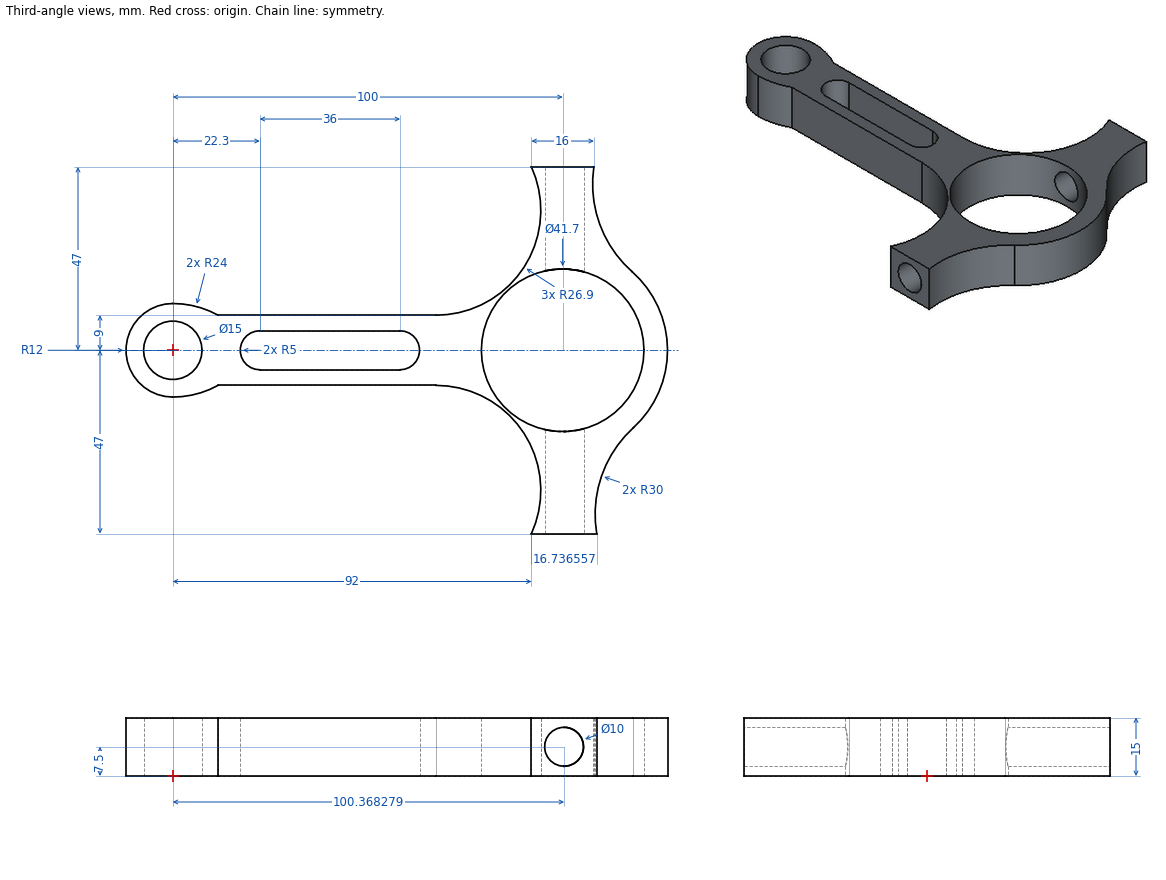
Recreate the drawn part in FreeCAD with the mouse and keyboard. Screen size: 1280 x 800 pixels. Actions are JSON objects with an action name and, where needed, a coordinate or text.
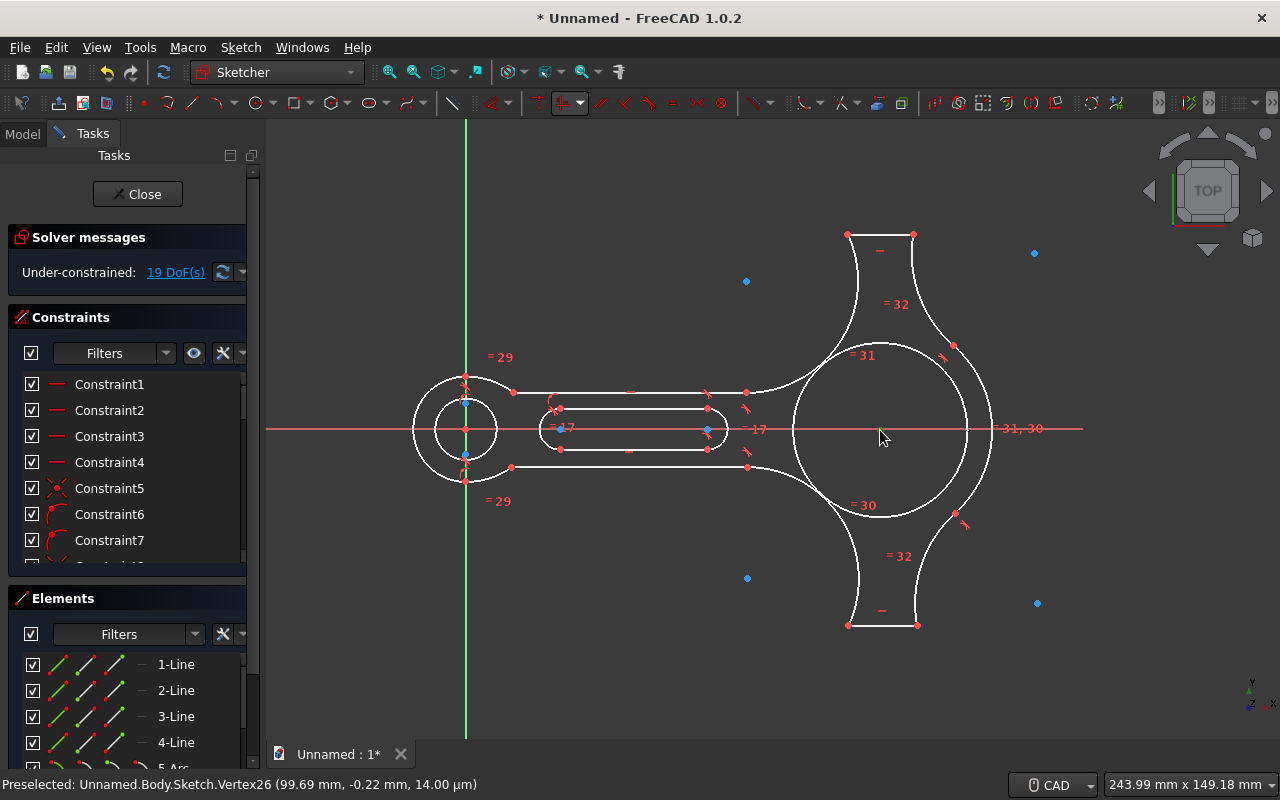
{"action": "left_click", "coordinate": [353, 429]}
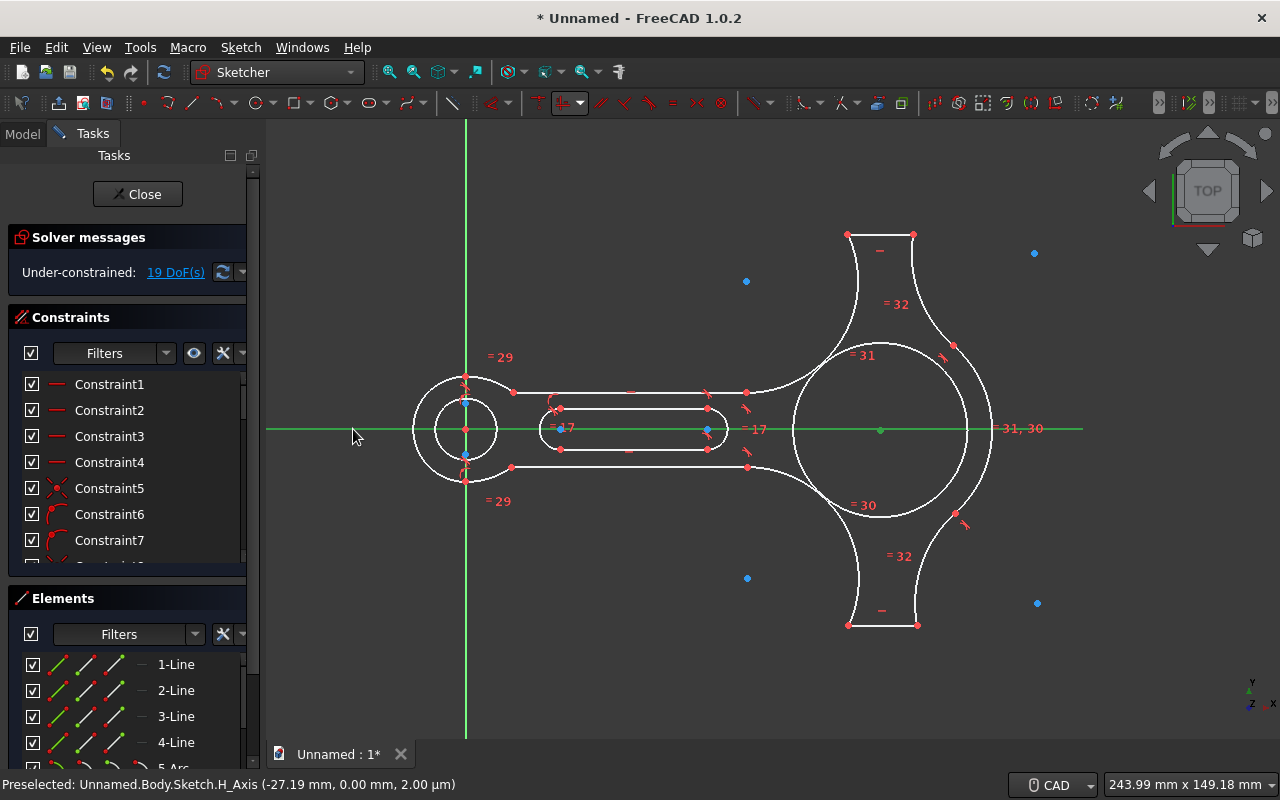
{"action": "left_click", "coordinate": [538, 104]}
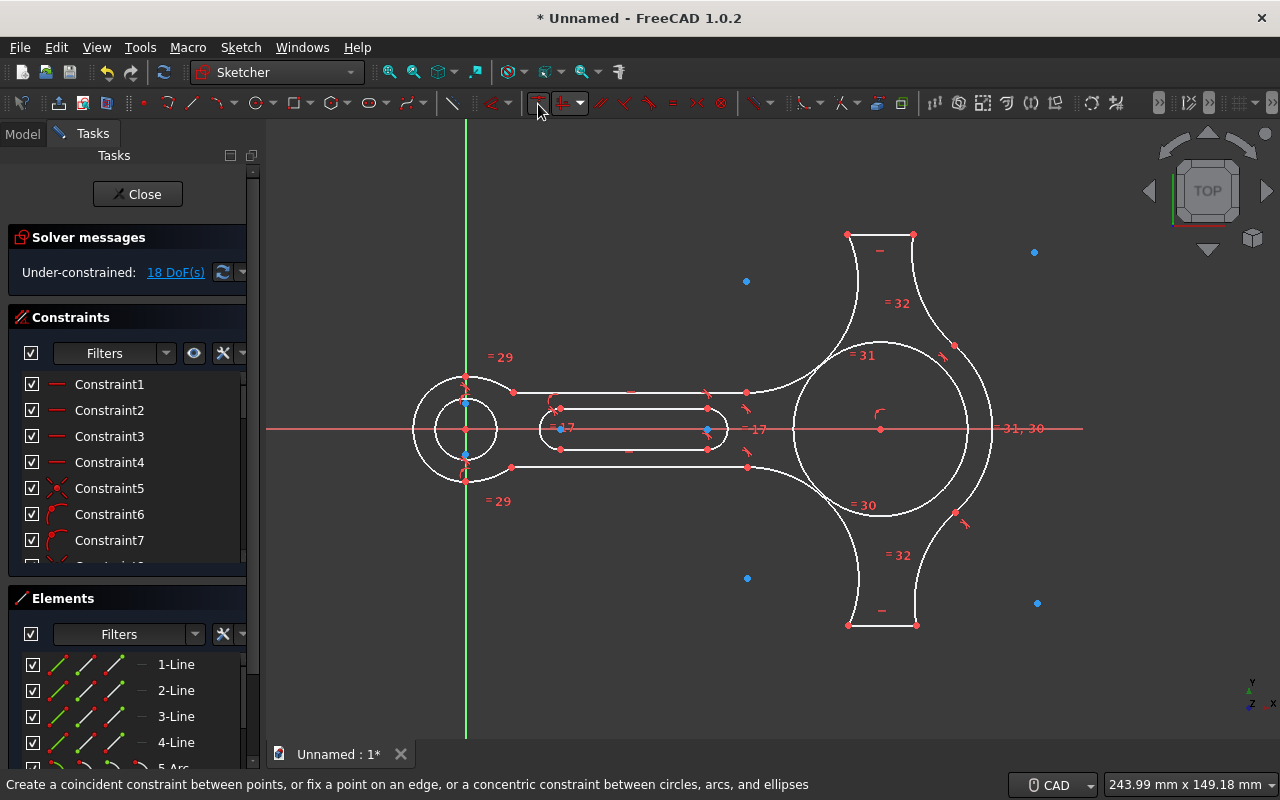
{"action": "left_click", "coordinate": [747, 579]}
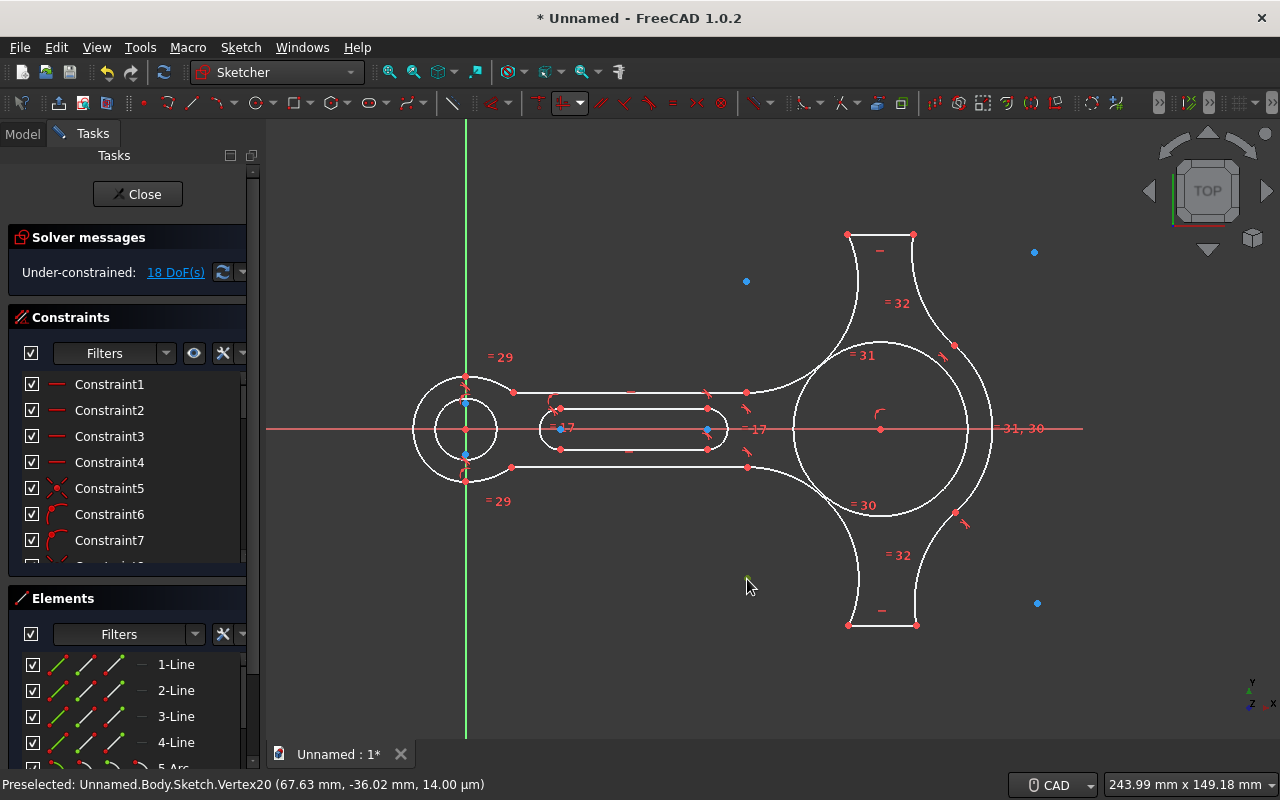
{"action": "left_click", "coordinate": [746, 281]}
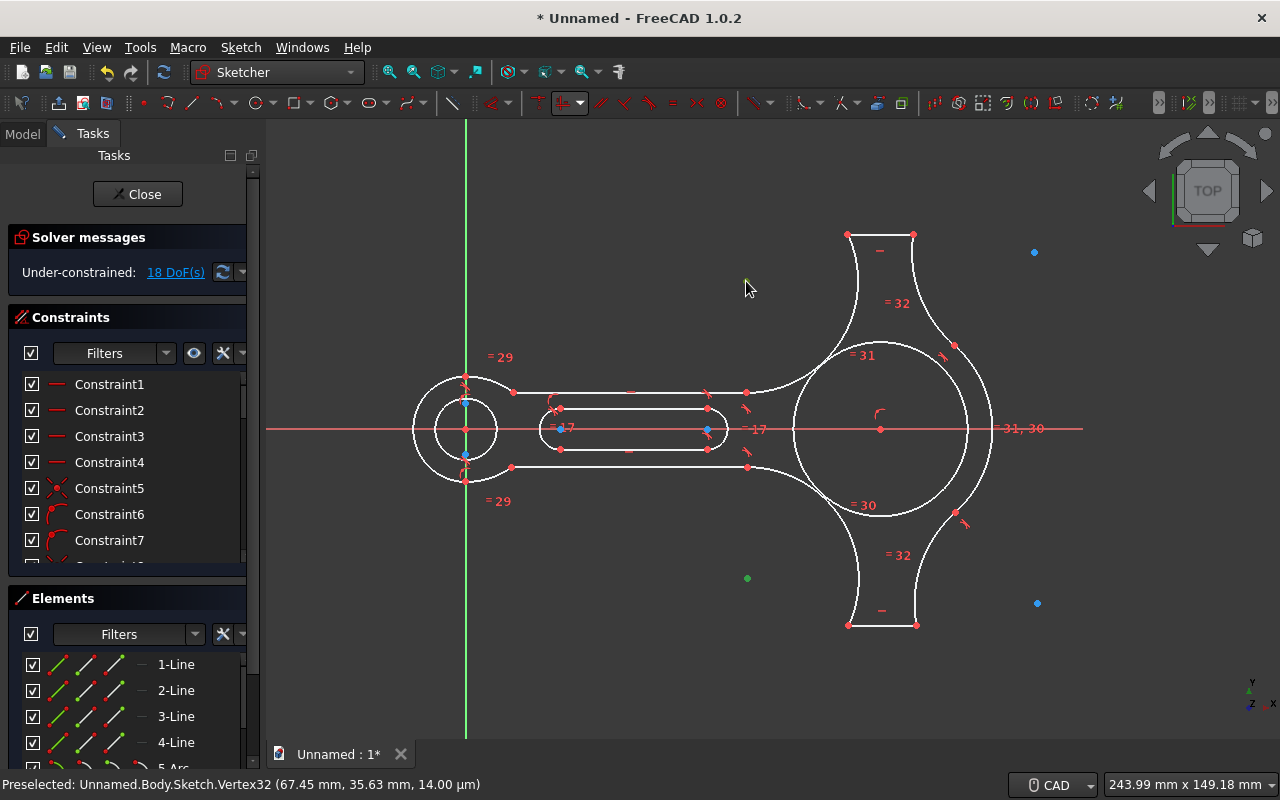
{"action": "left_click", "coordinate": [353, 429]}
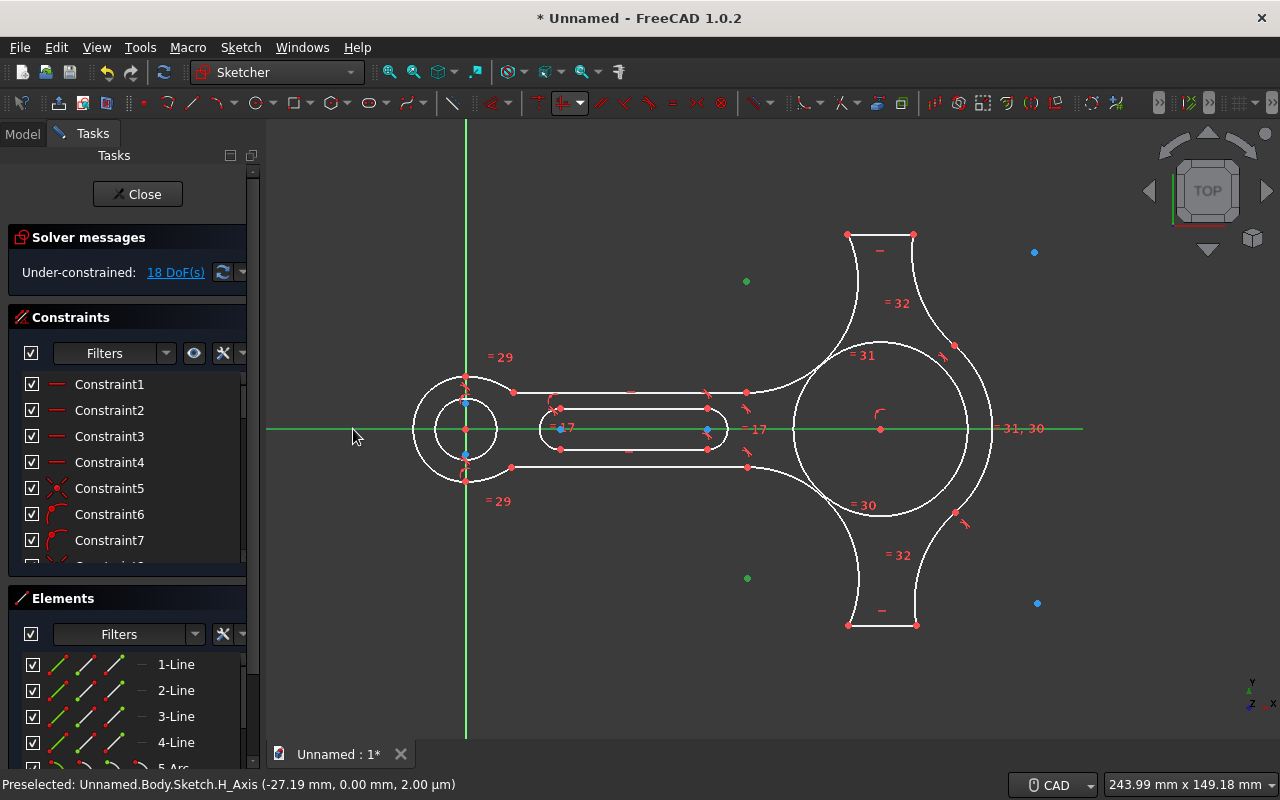
{"action": "left_click", "coordinate": [698, 104]}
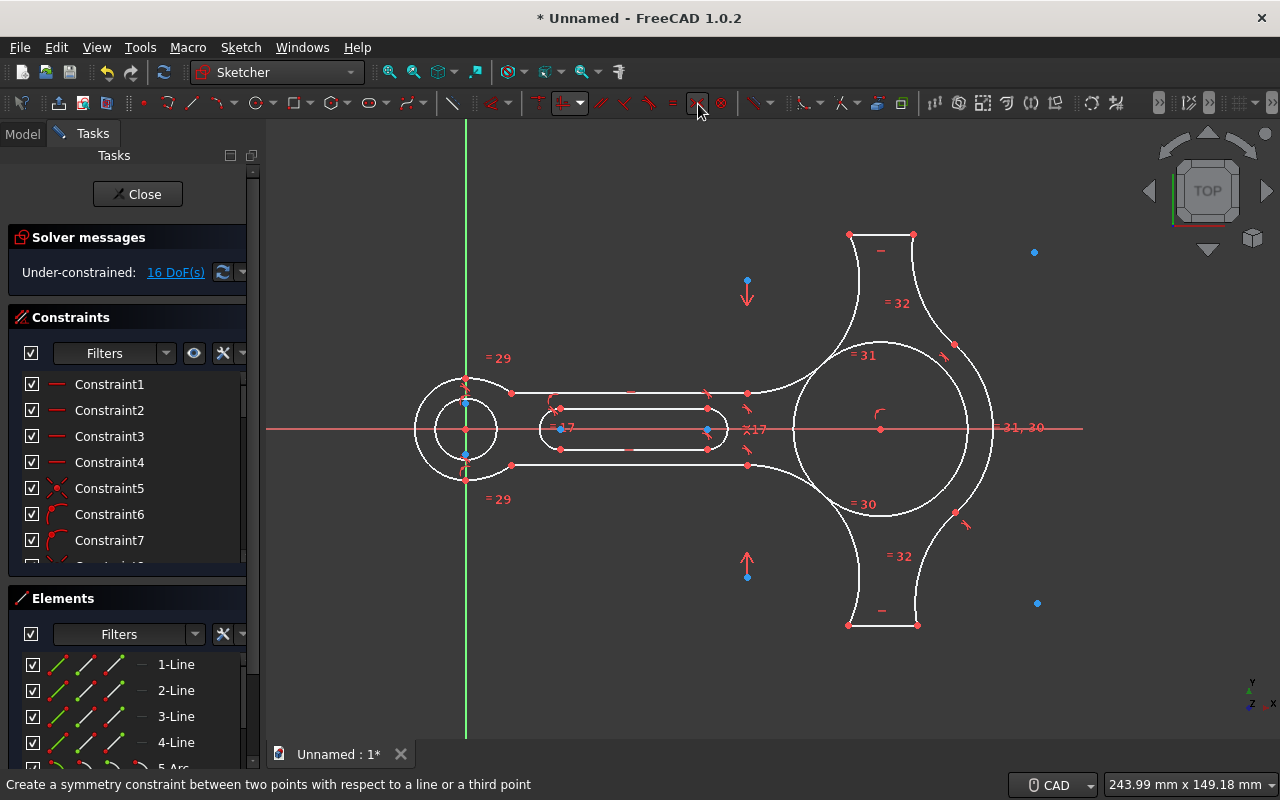
{"action": "left_click", "coordinate": [492, 104]}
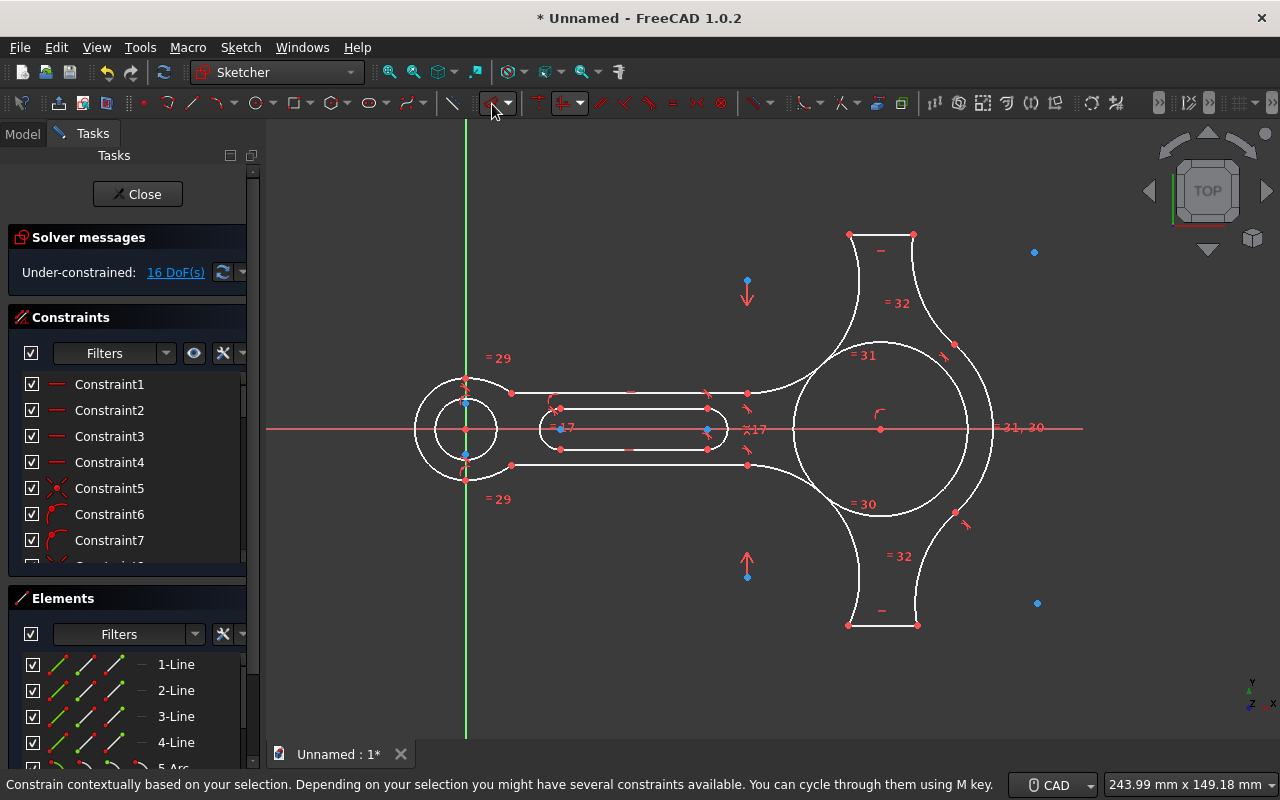
{"action": "left_click", "coordinate": [499, 386]}
{"action": "left_click", "coordinate": [513, 357]}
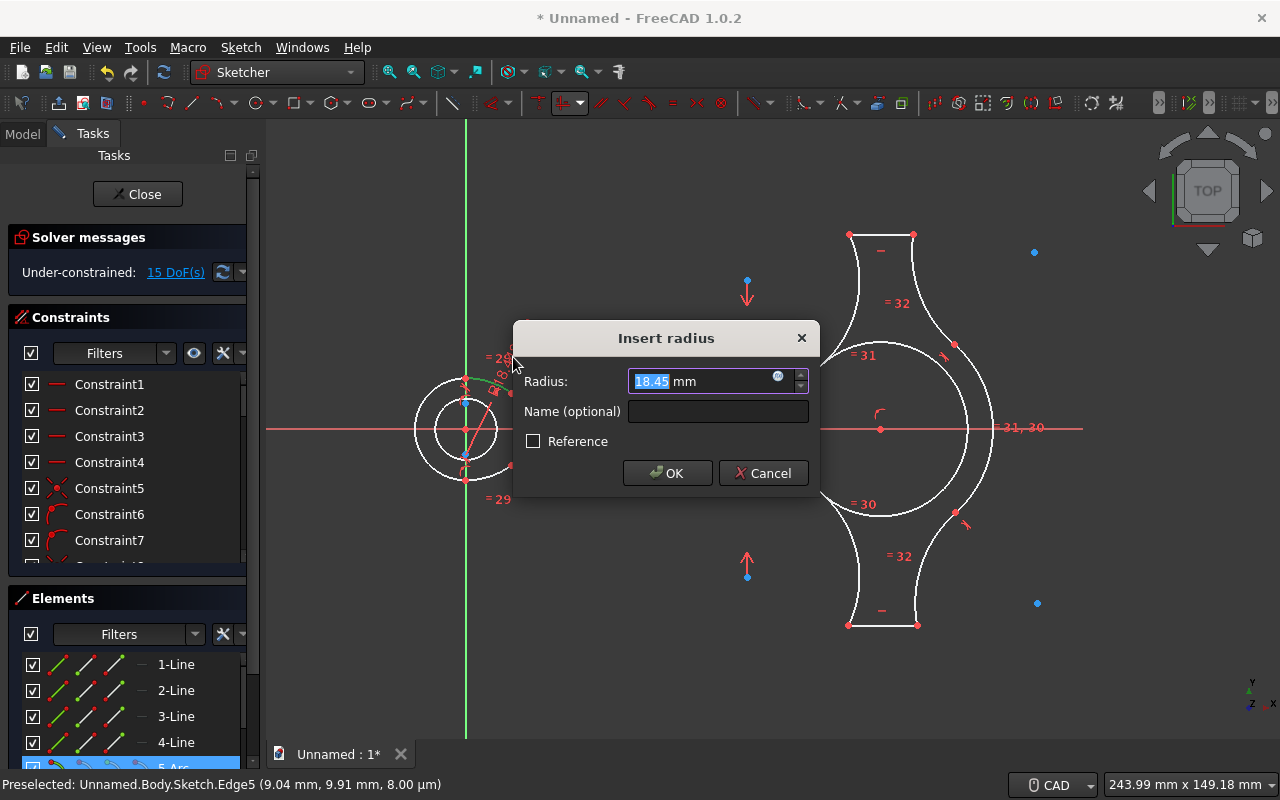
{"action": "type", "text": "24"}
{"action": "key", "text": "Return"}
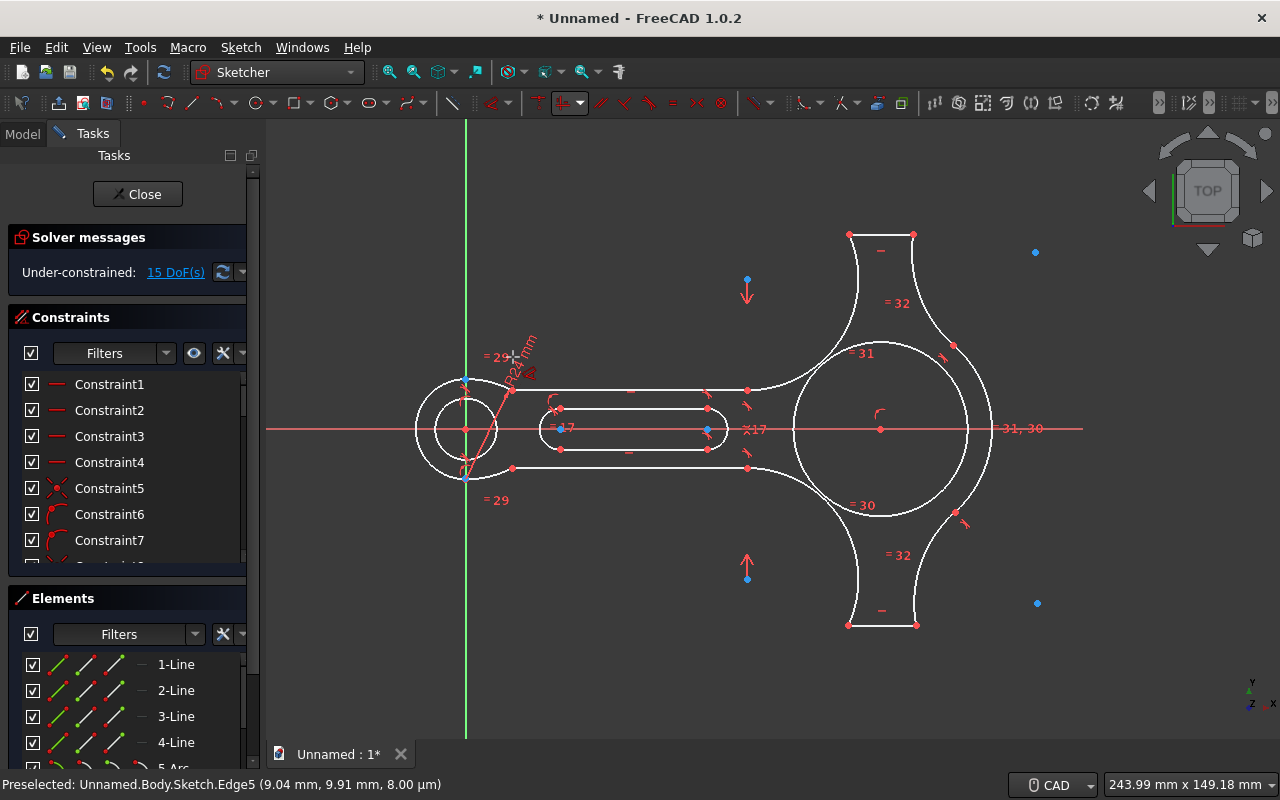
{"action": "left_click", "coordinate": [425, 400]}
{"action": "left_click", "coordinate": [399, 381]}